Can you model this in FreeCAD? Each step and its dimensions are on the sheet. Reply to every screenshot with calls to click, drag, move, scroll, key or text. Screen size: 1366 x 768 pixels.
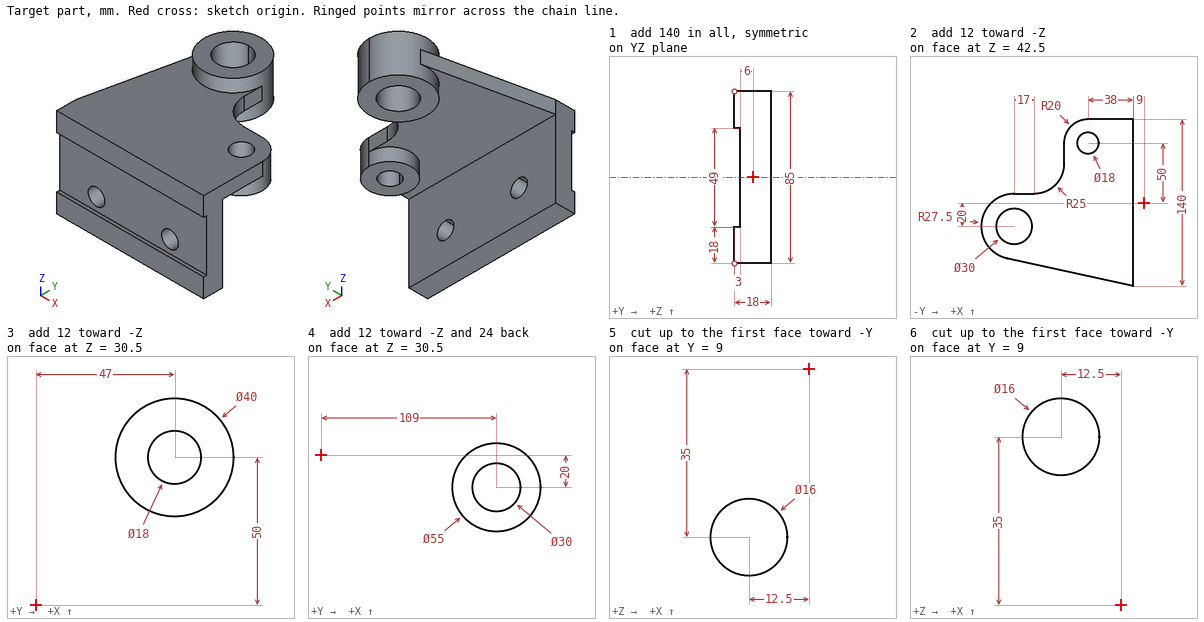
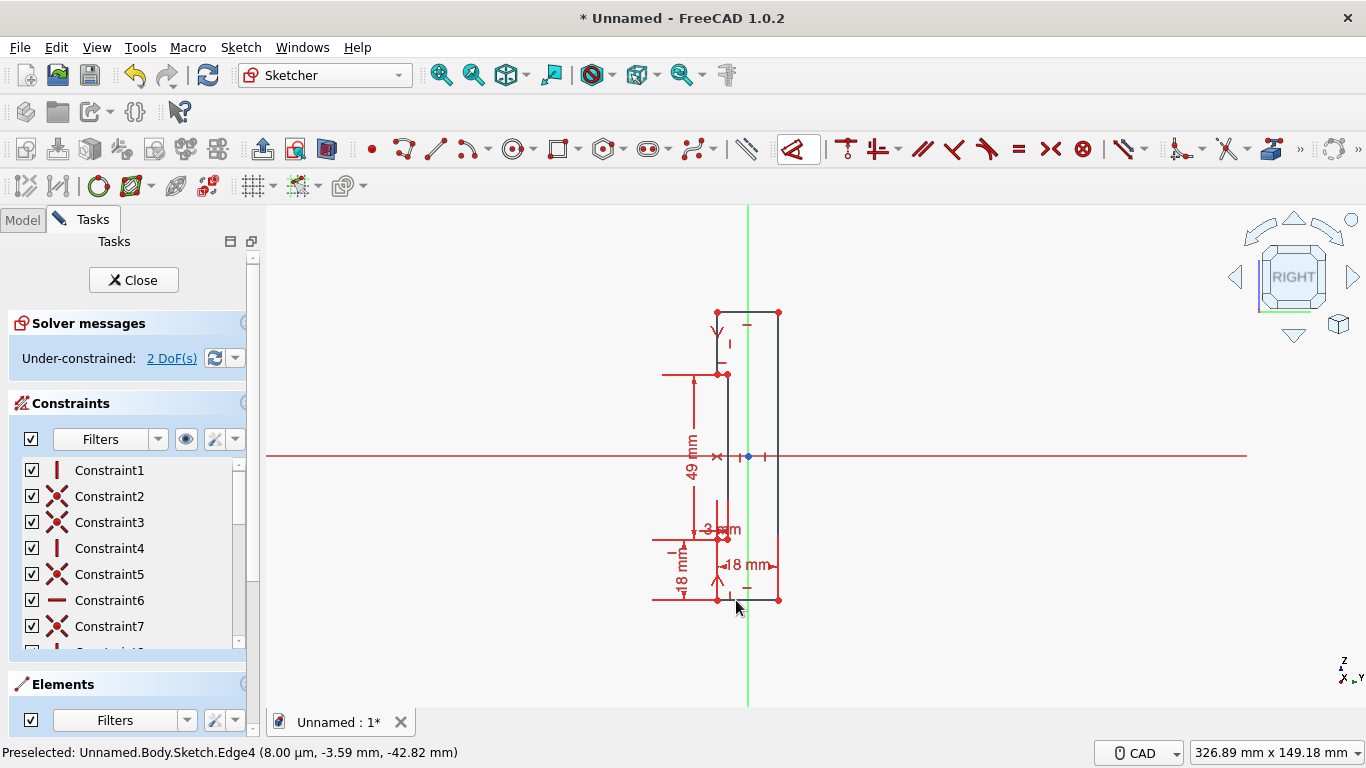
click(778, 514)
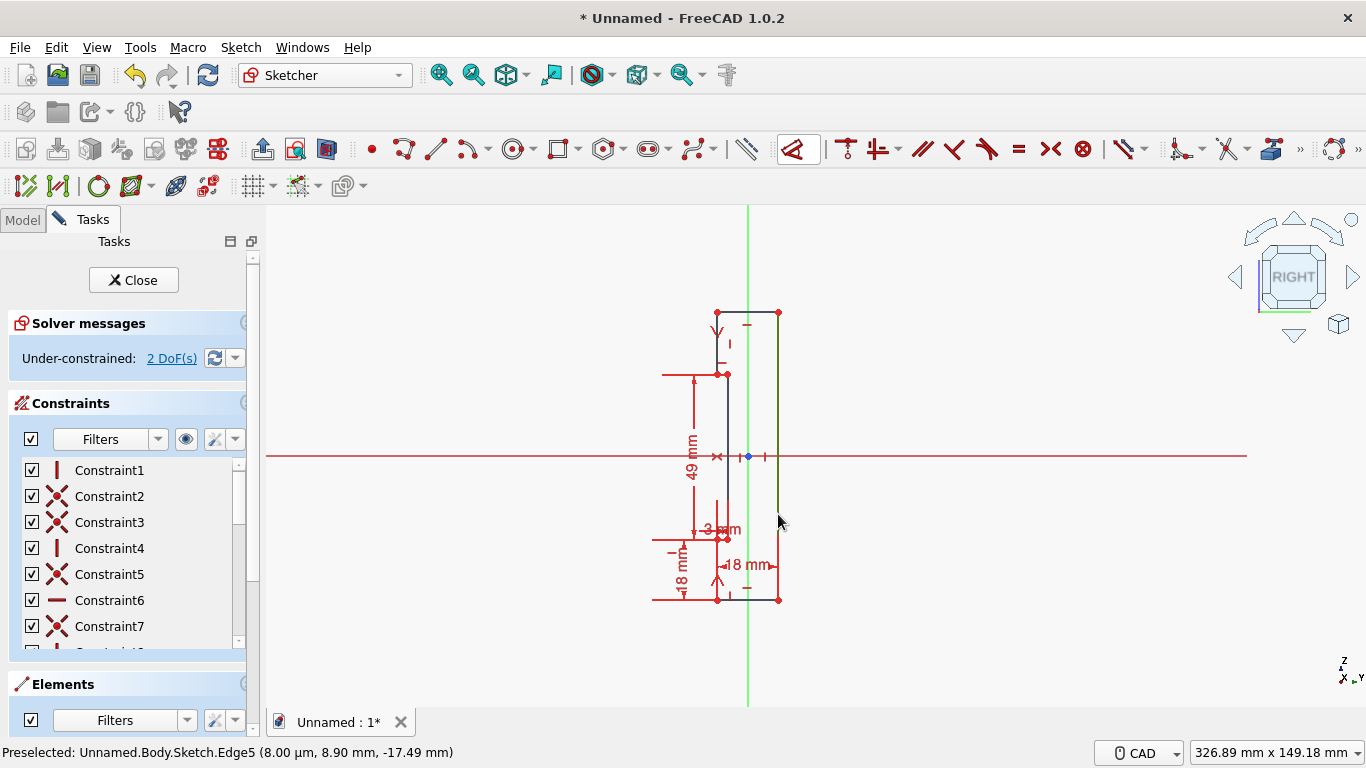
key(i)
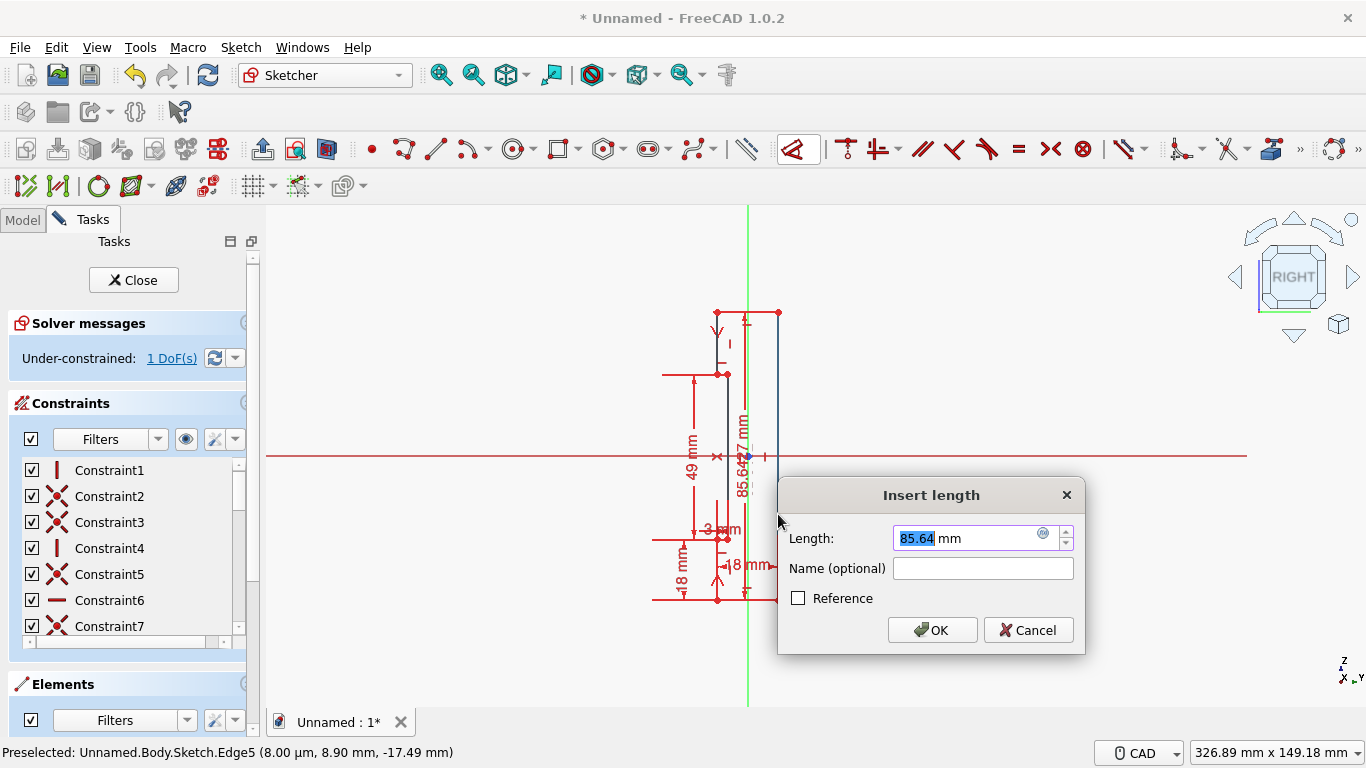
text(85)
key(Return)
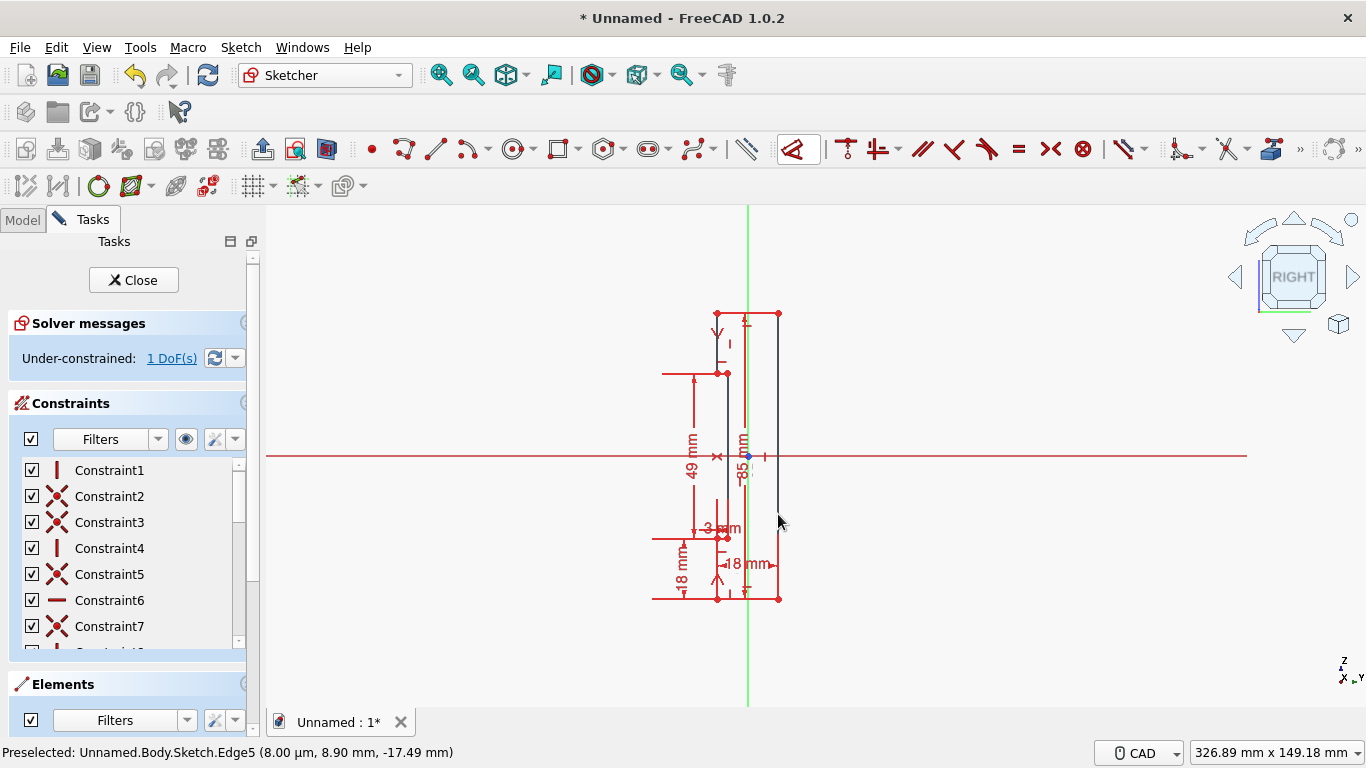
scroll(728, 374, up, 4)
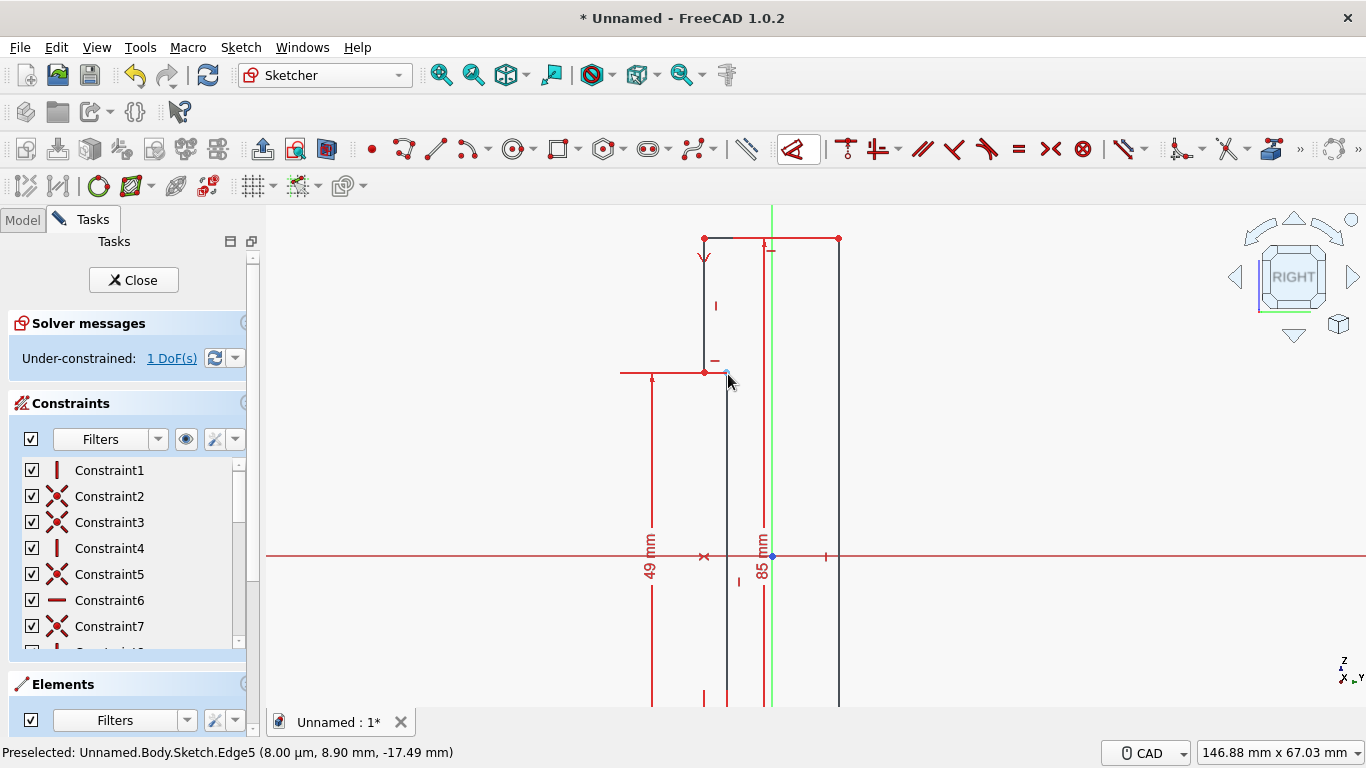
click(727, 373)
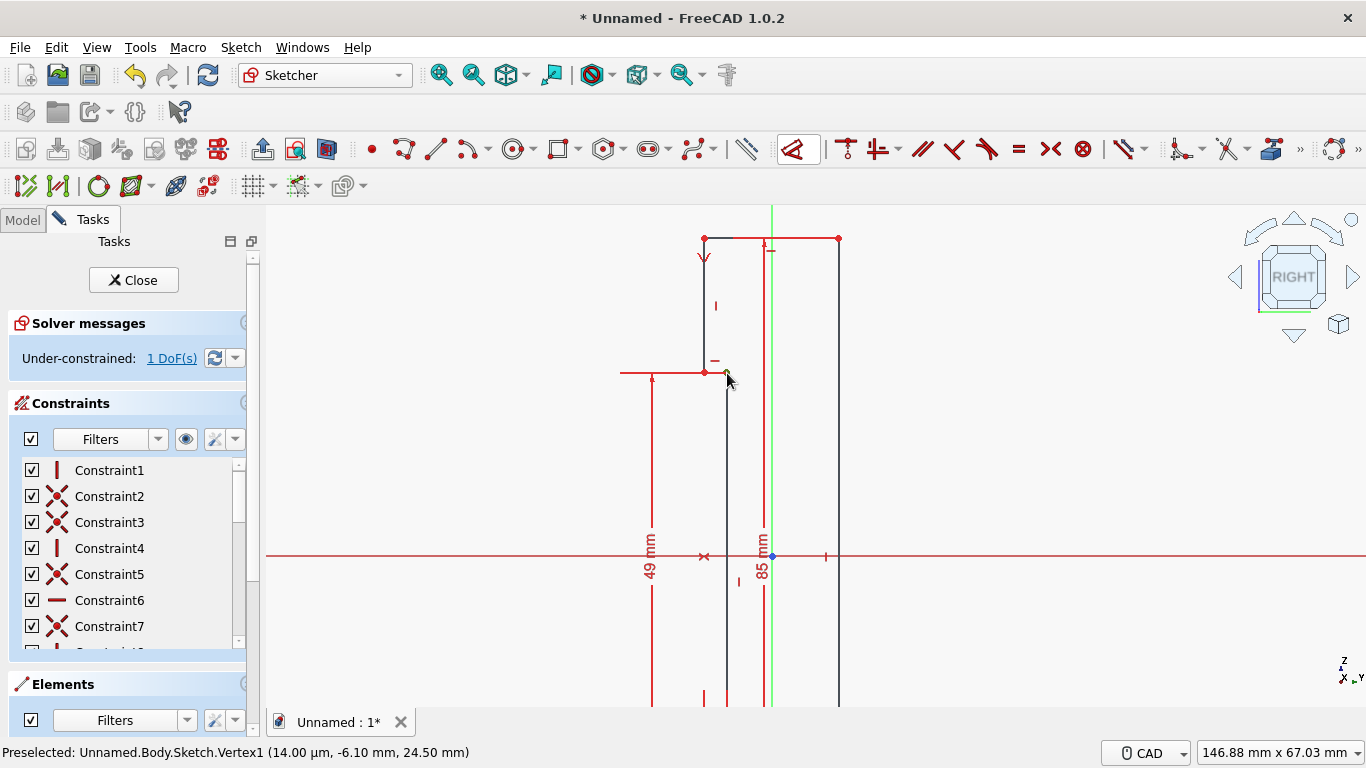
click(814, 150)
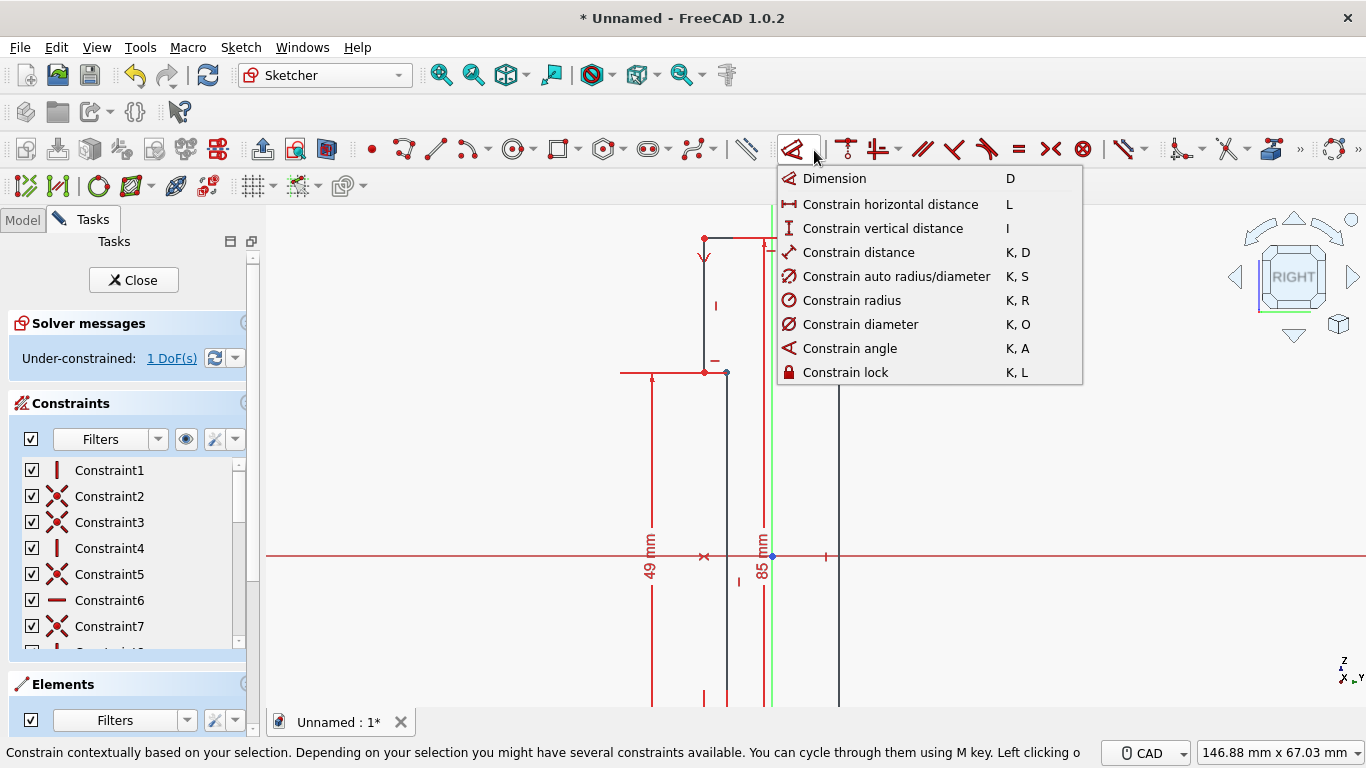
click(930, 204)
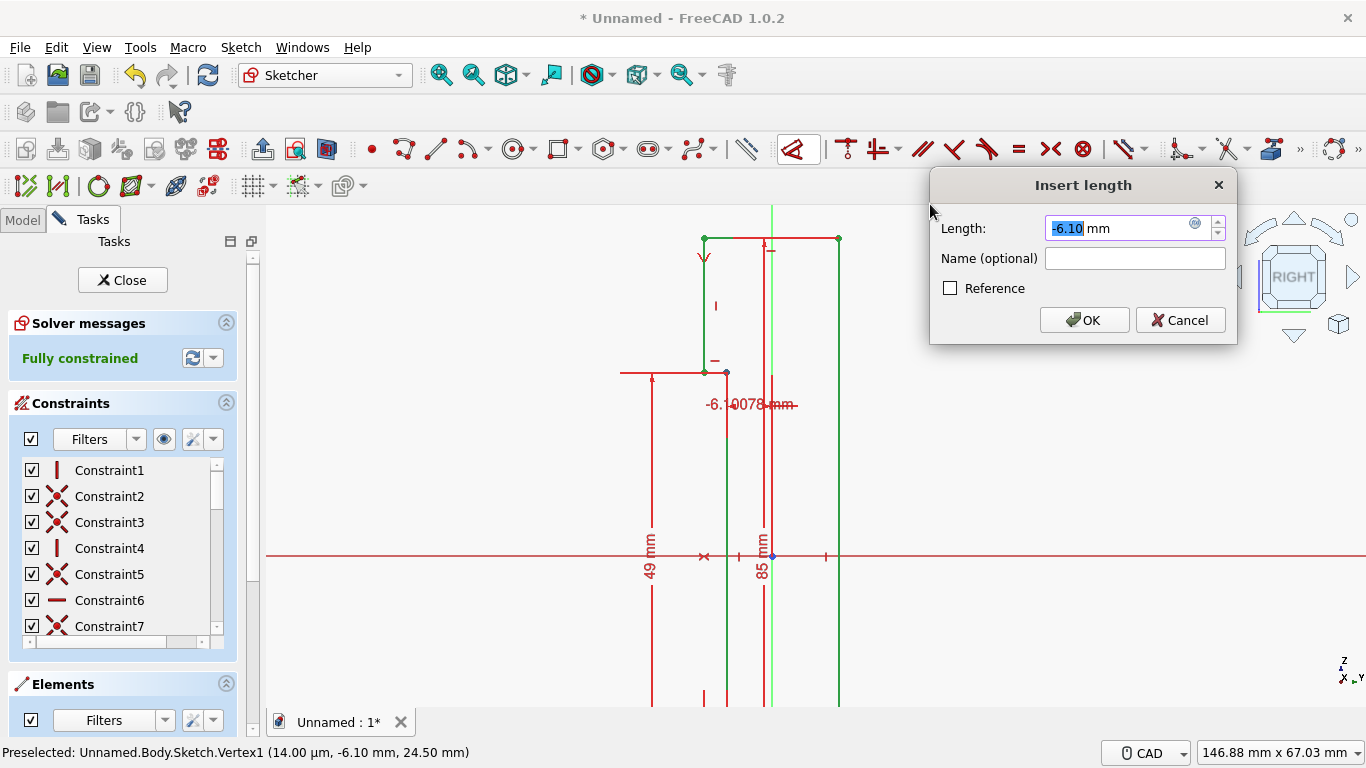
text(-6)
key(Return)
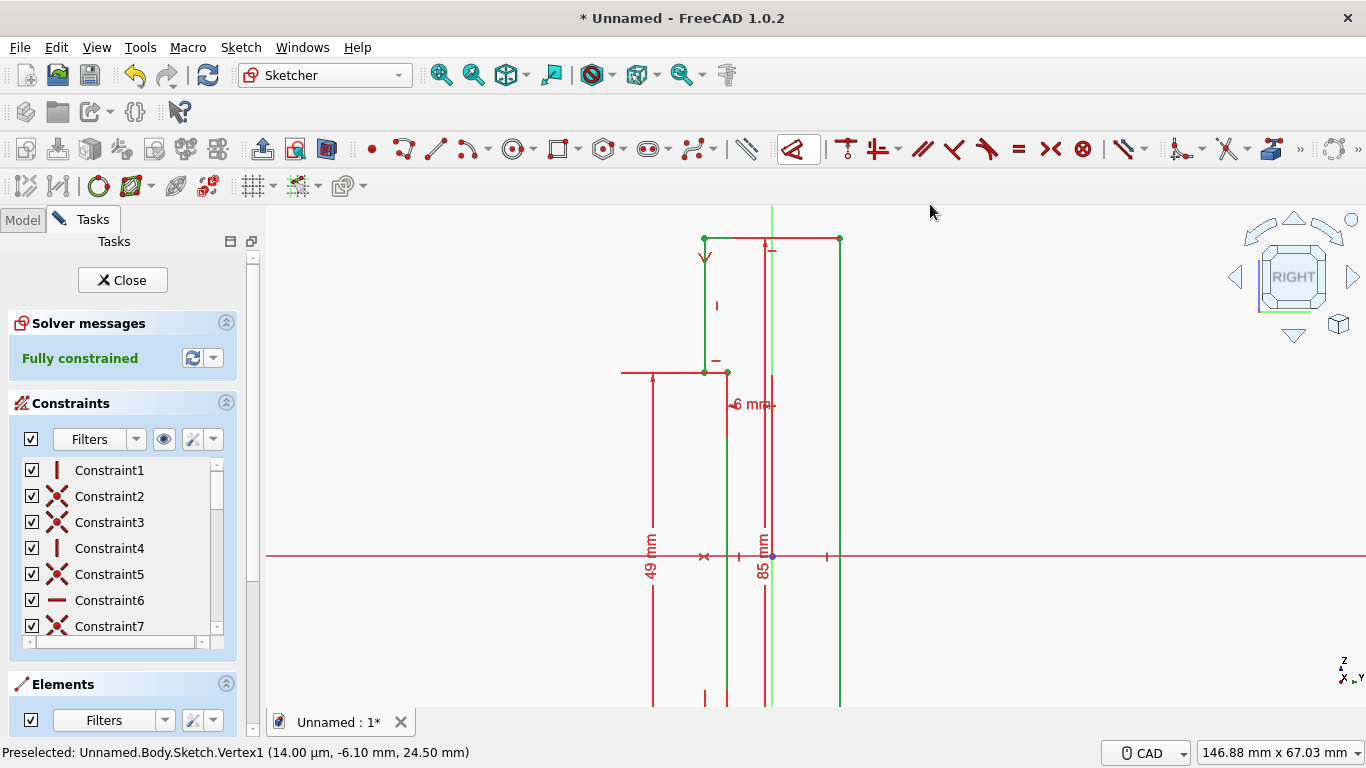
click(123, 280)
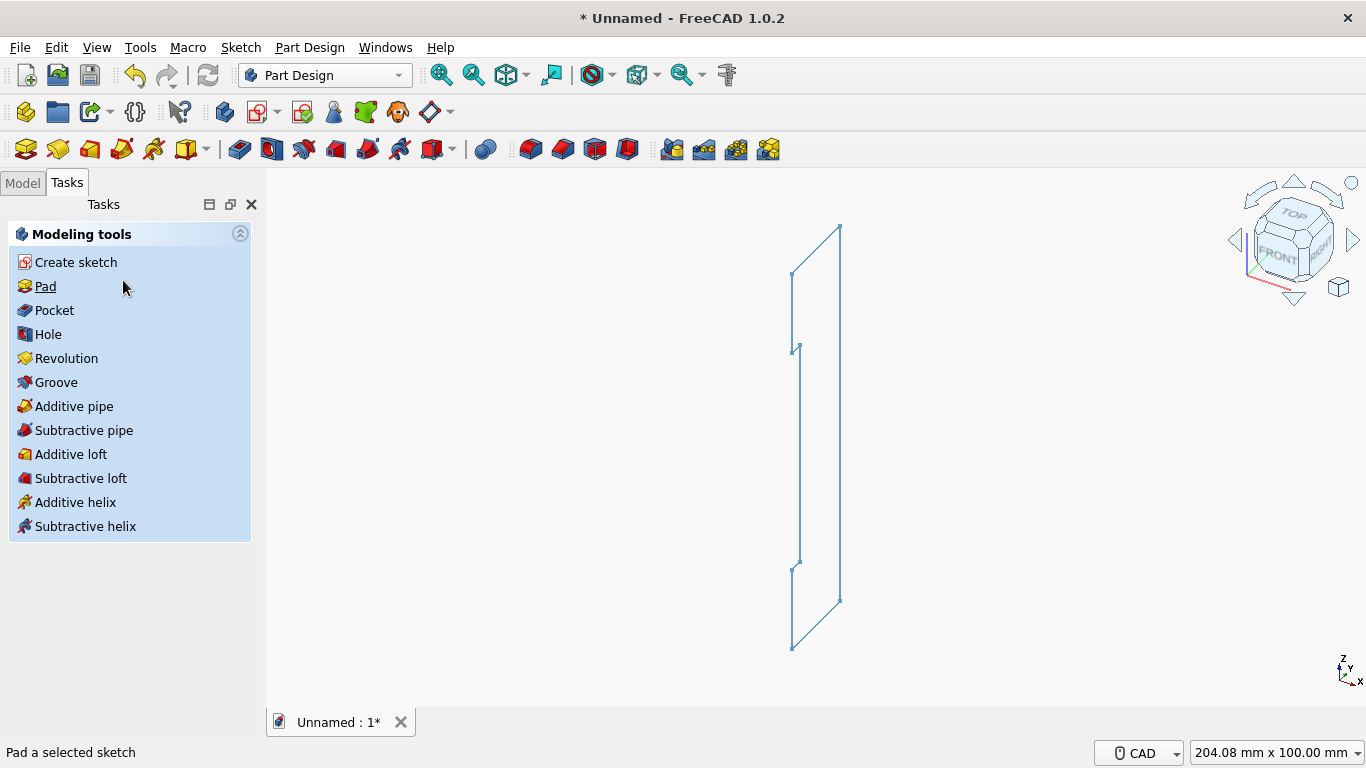
click(26, 150)